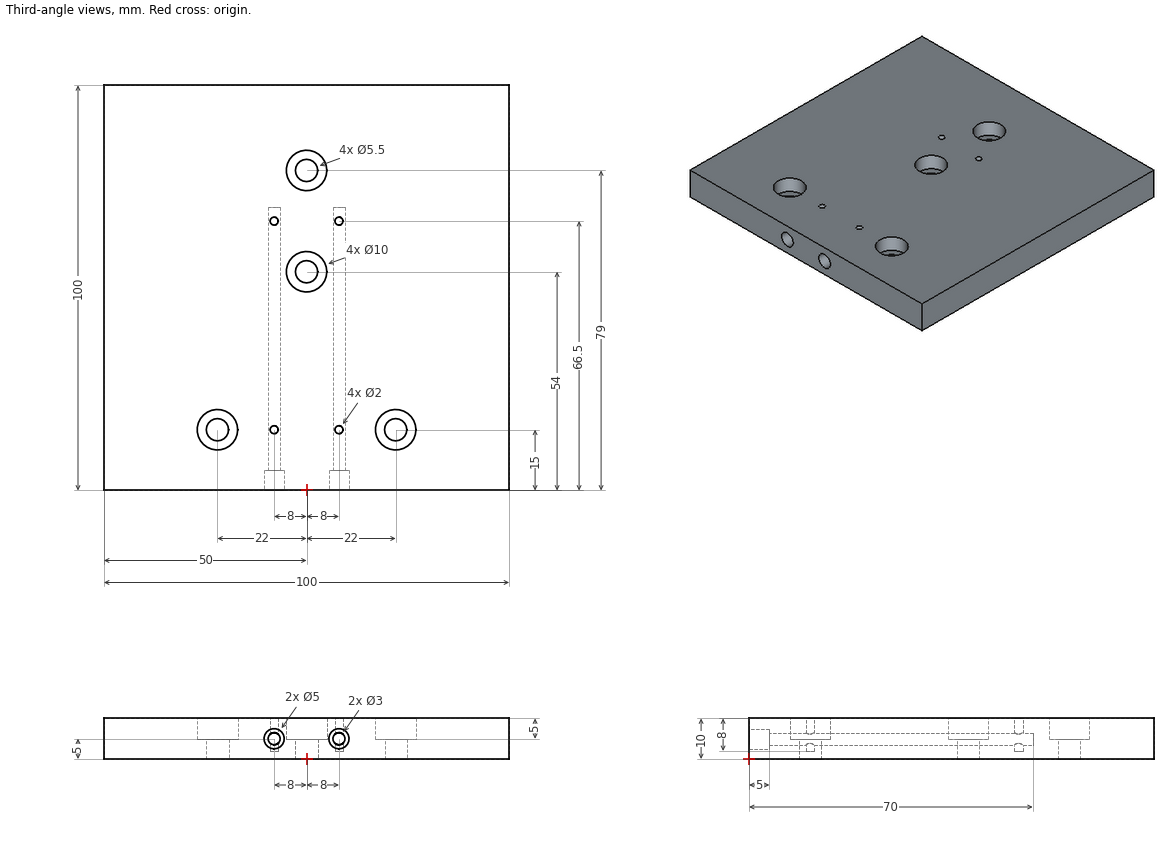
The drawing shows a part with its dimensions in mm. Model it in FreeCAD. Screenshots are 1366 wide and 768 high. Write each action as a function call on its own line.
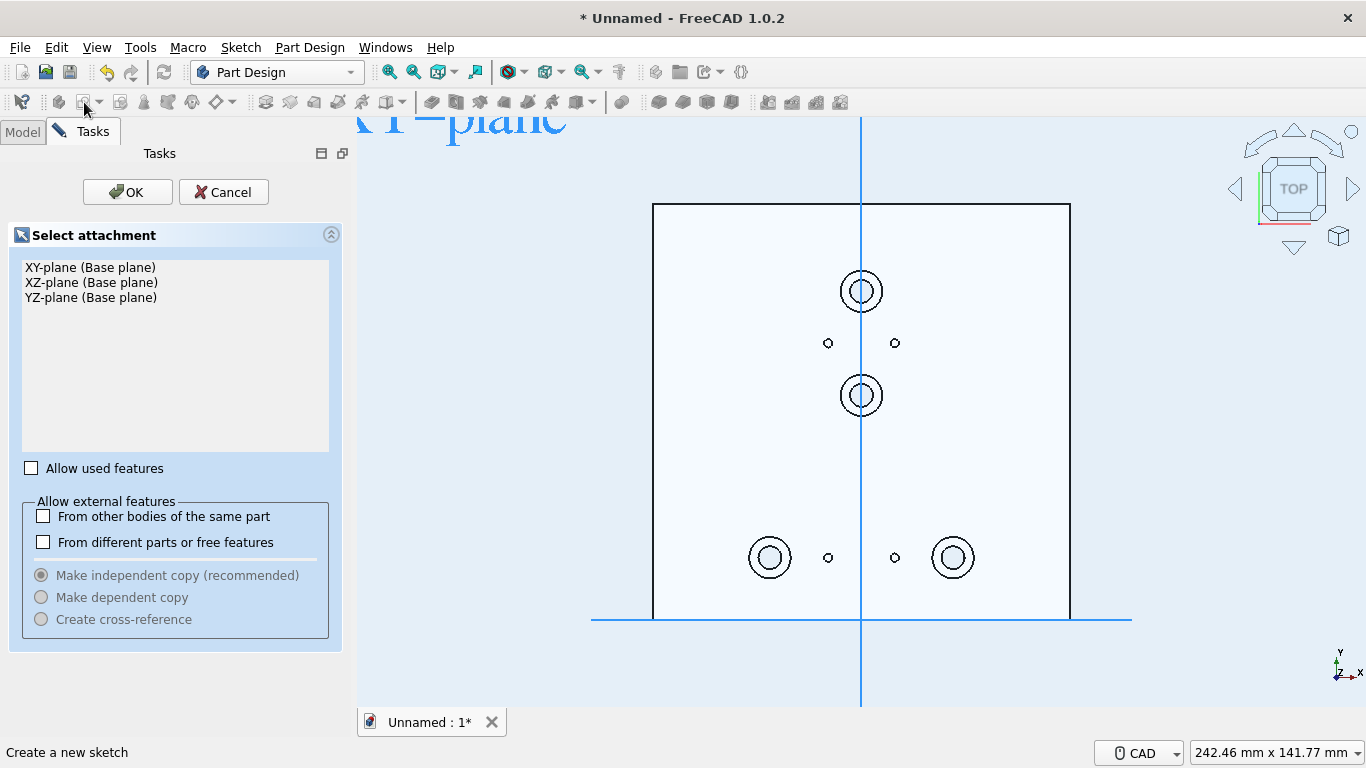
click(82, 282)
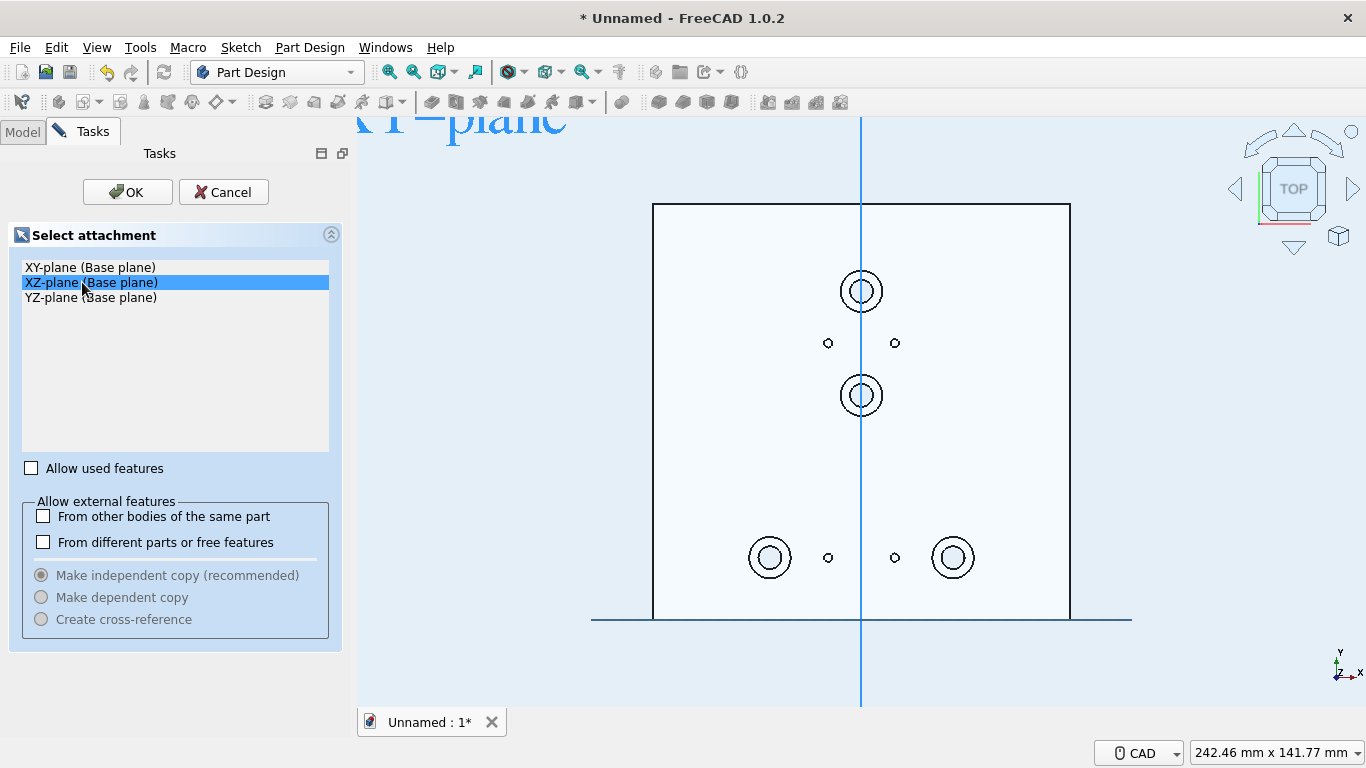
click(128, 192)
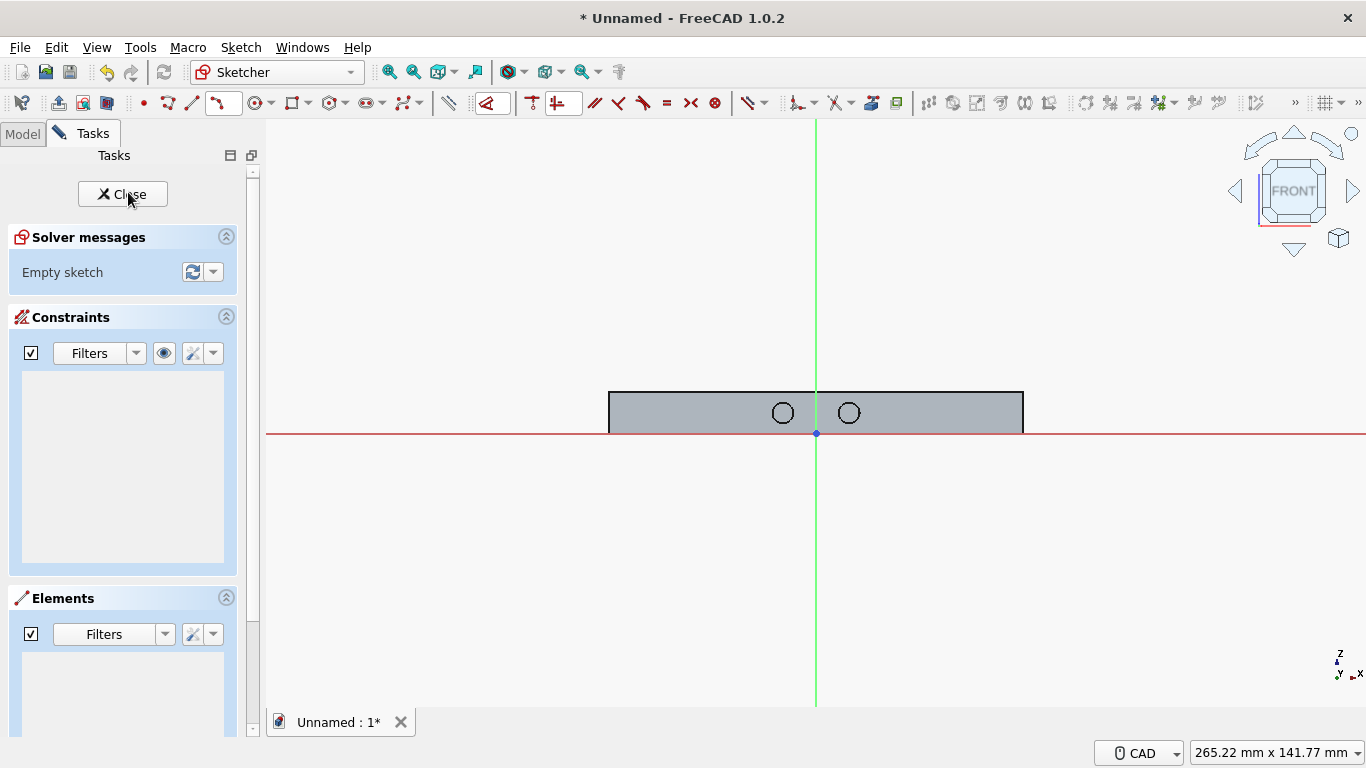
scroll(827, 421, up, 10)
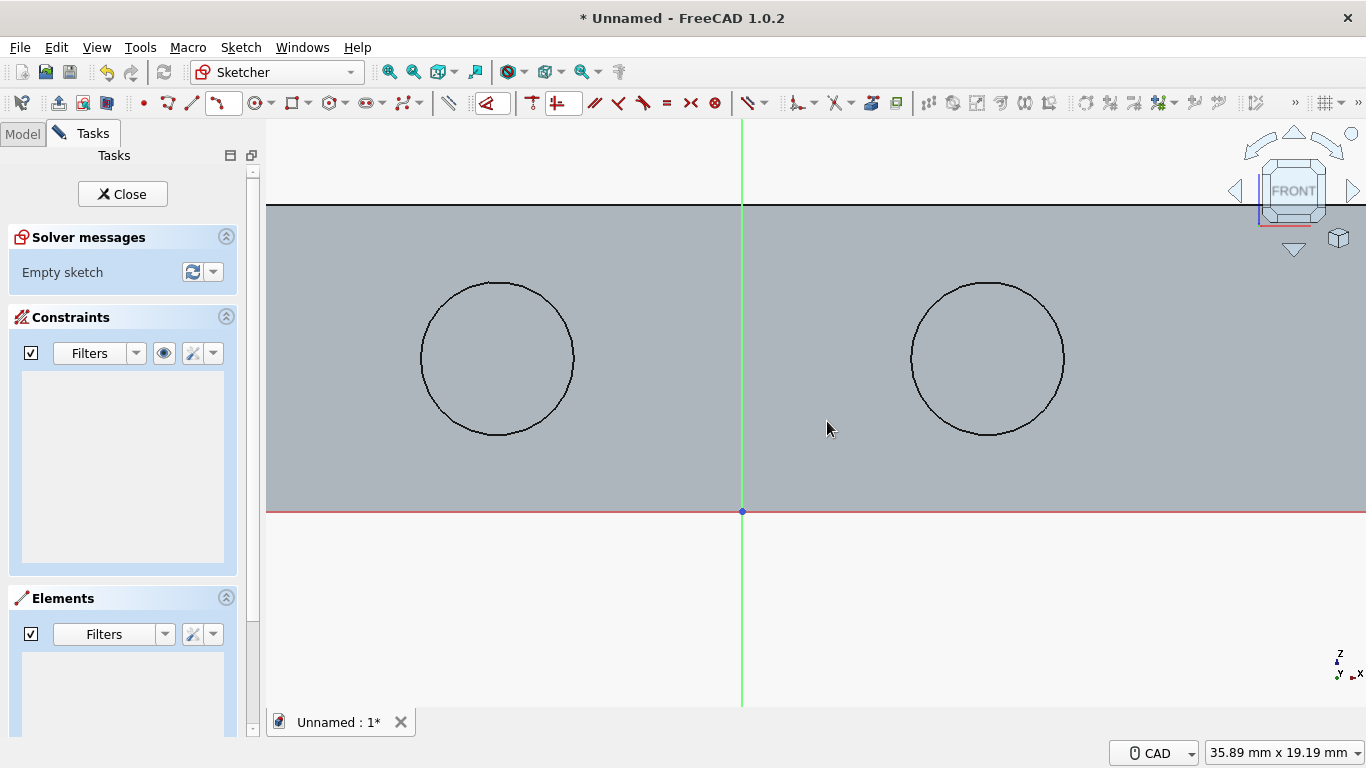
click(256, 104)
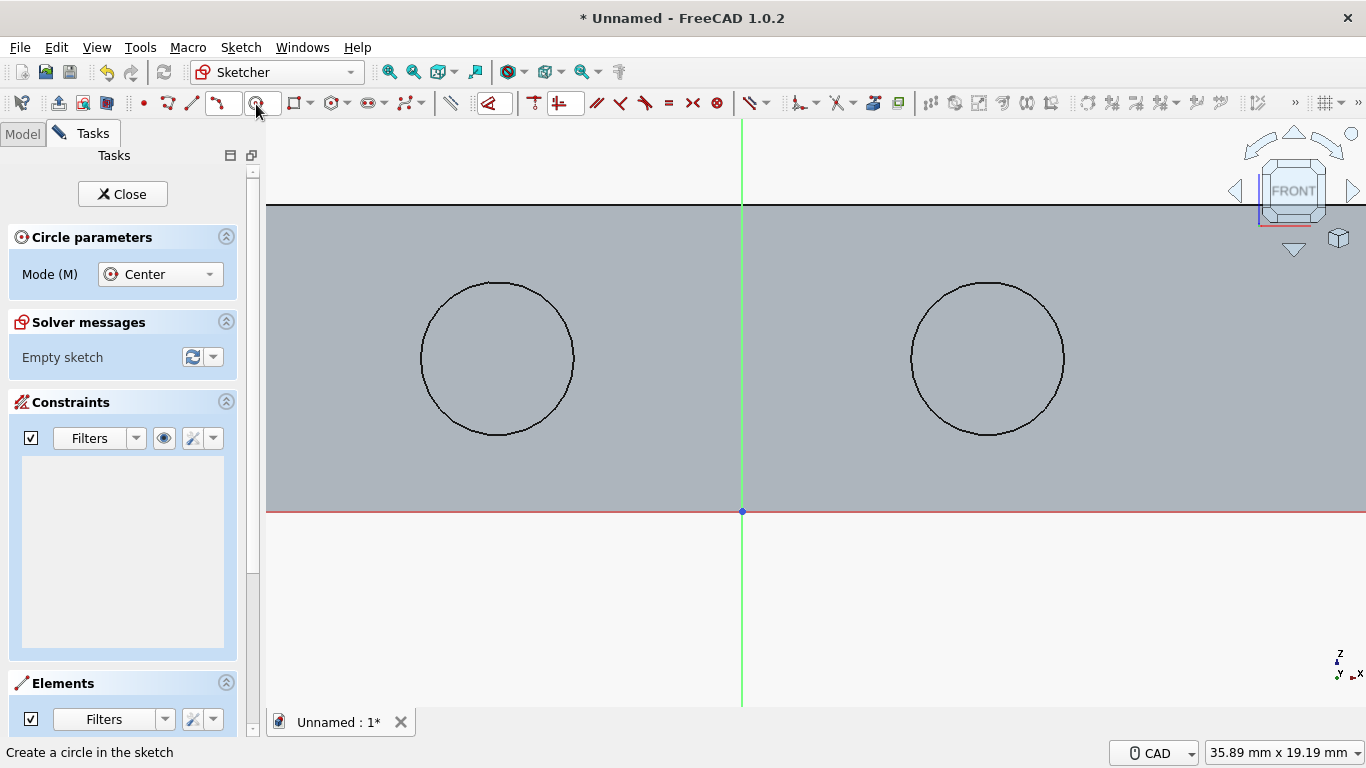
click(988, 359)
click(1020, 326)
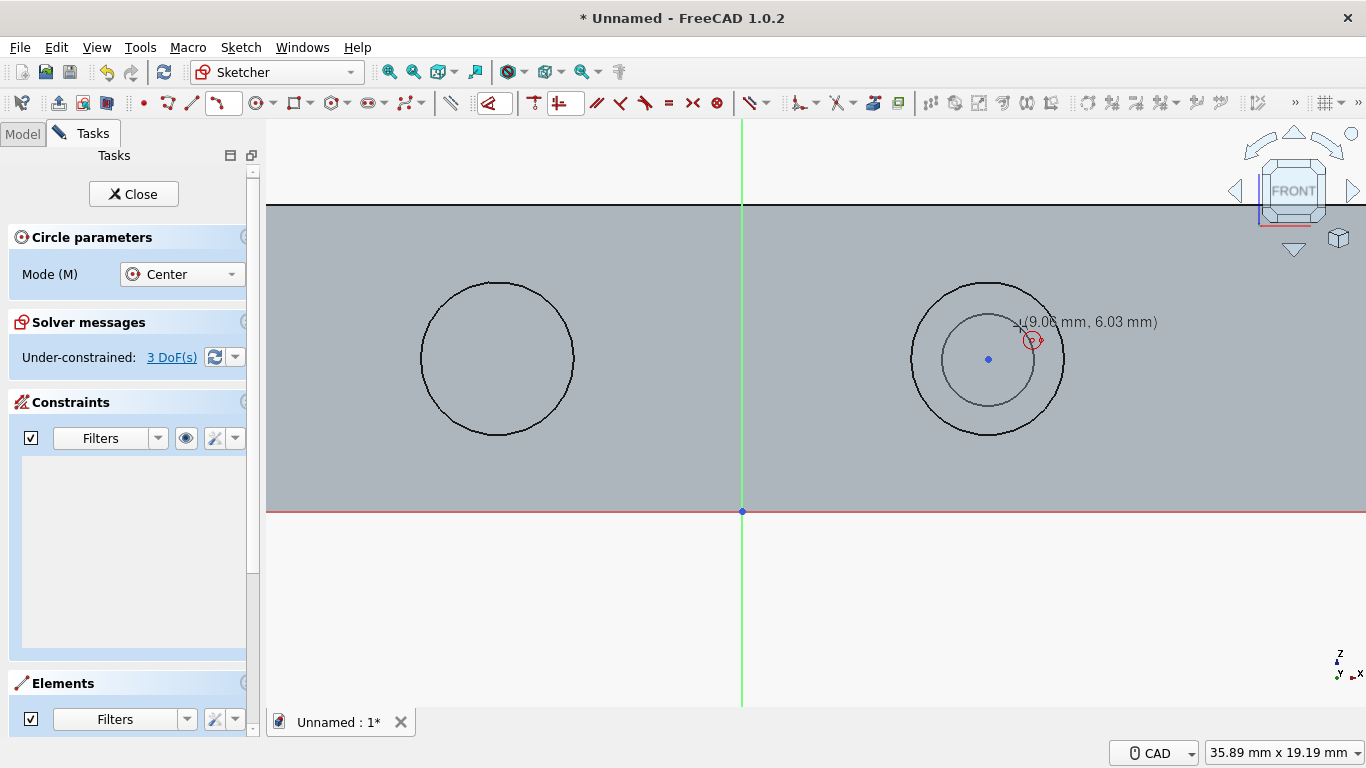
click(497, 359)
click(530, 326)
key(Escape)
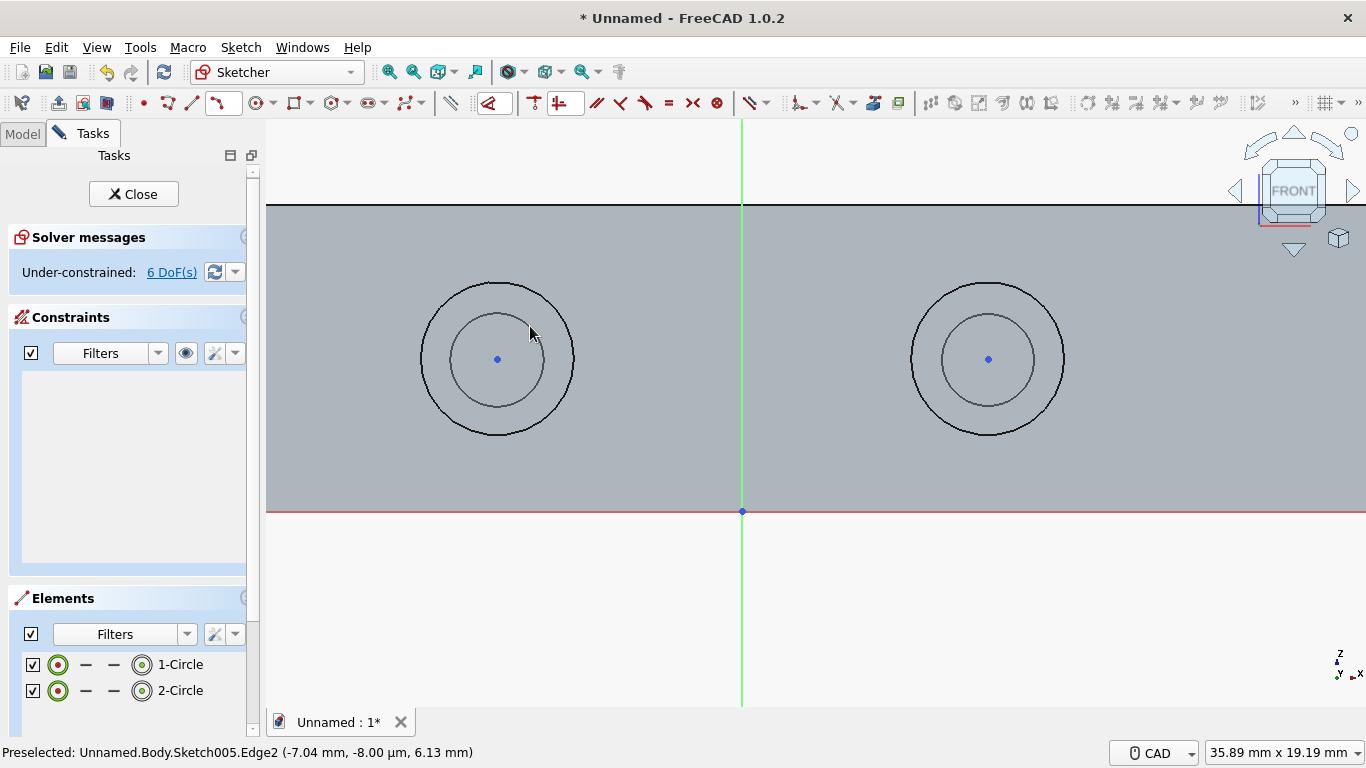
click(1020, 327)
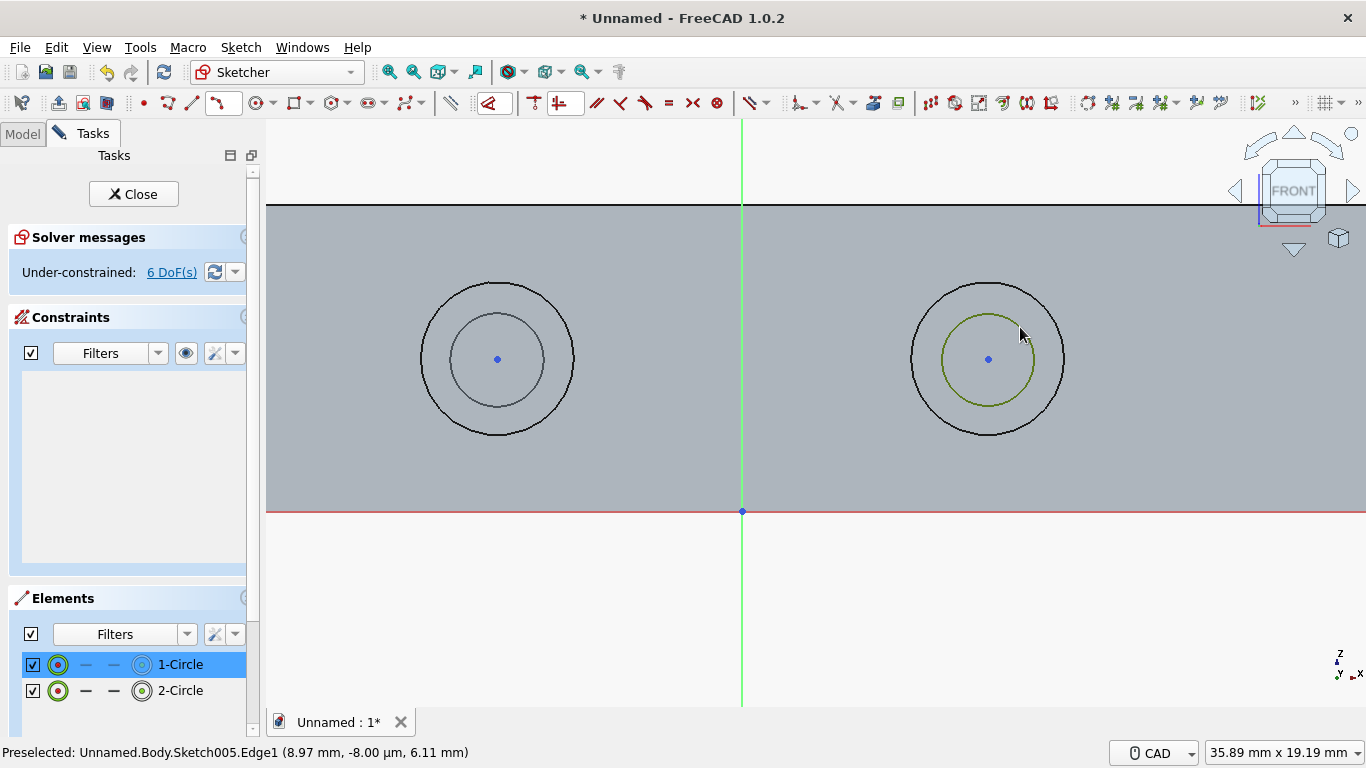
click(530, 327)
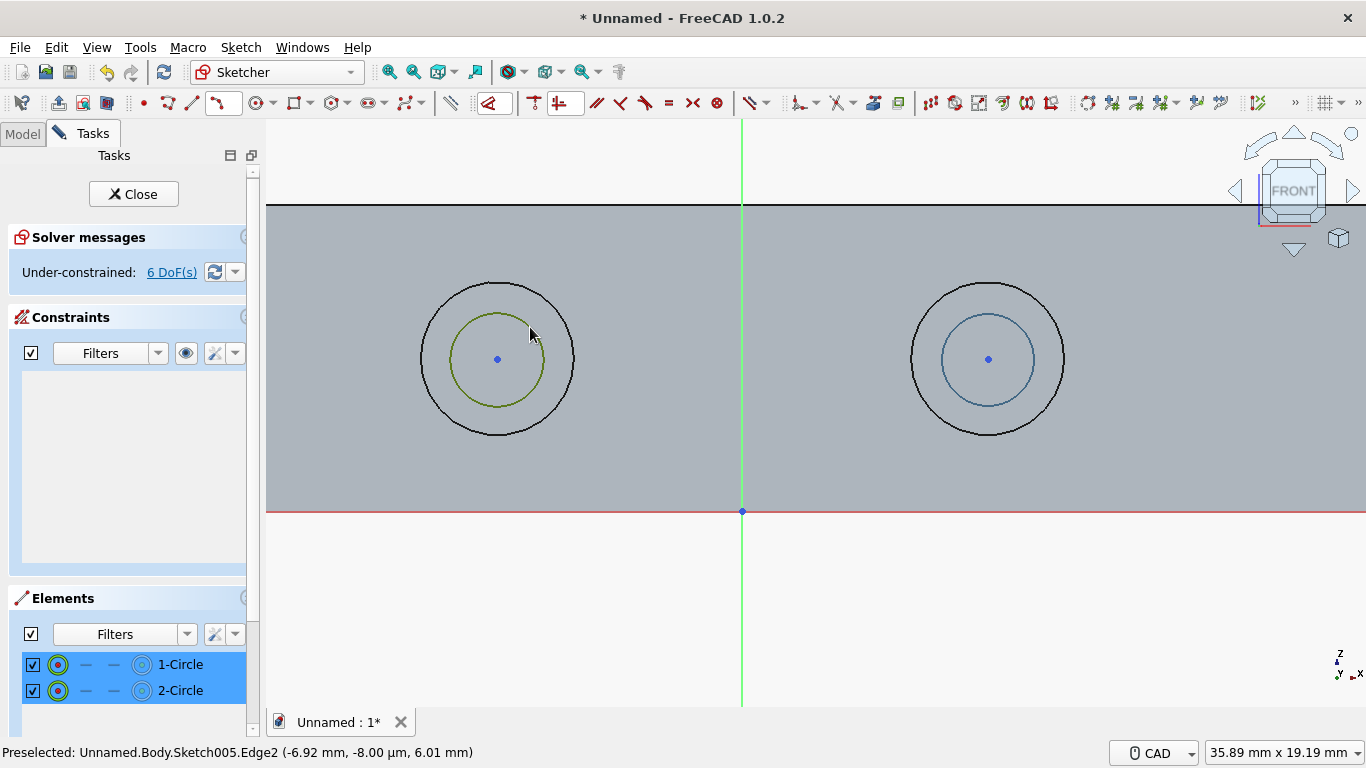
click(670, 104)